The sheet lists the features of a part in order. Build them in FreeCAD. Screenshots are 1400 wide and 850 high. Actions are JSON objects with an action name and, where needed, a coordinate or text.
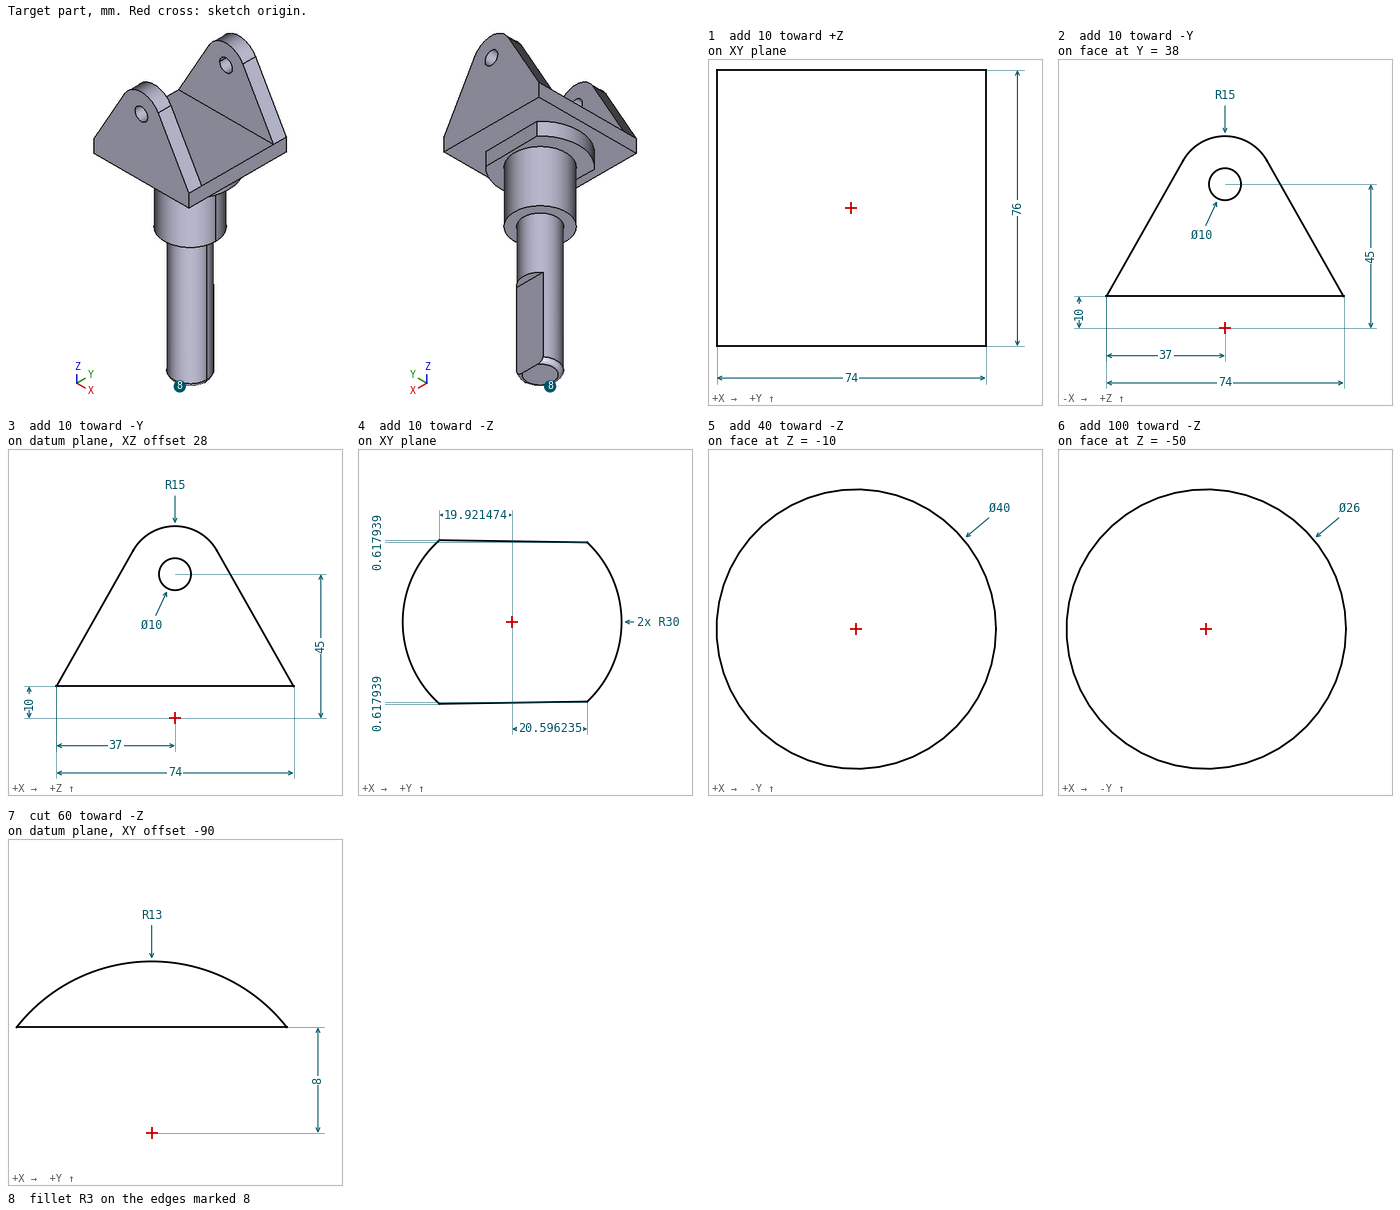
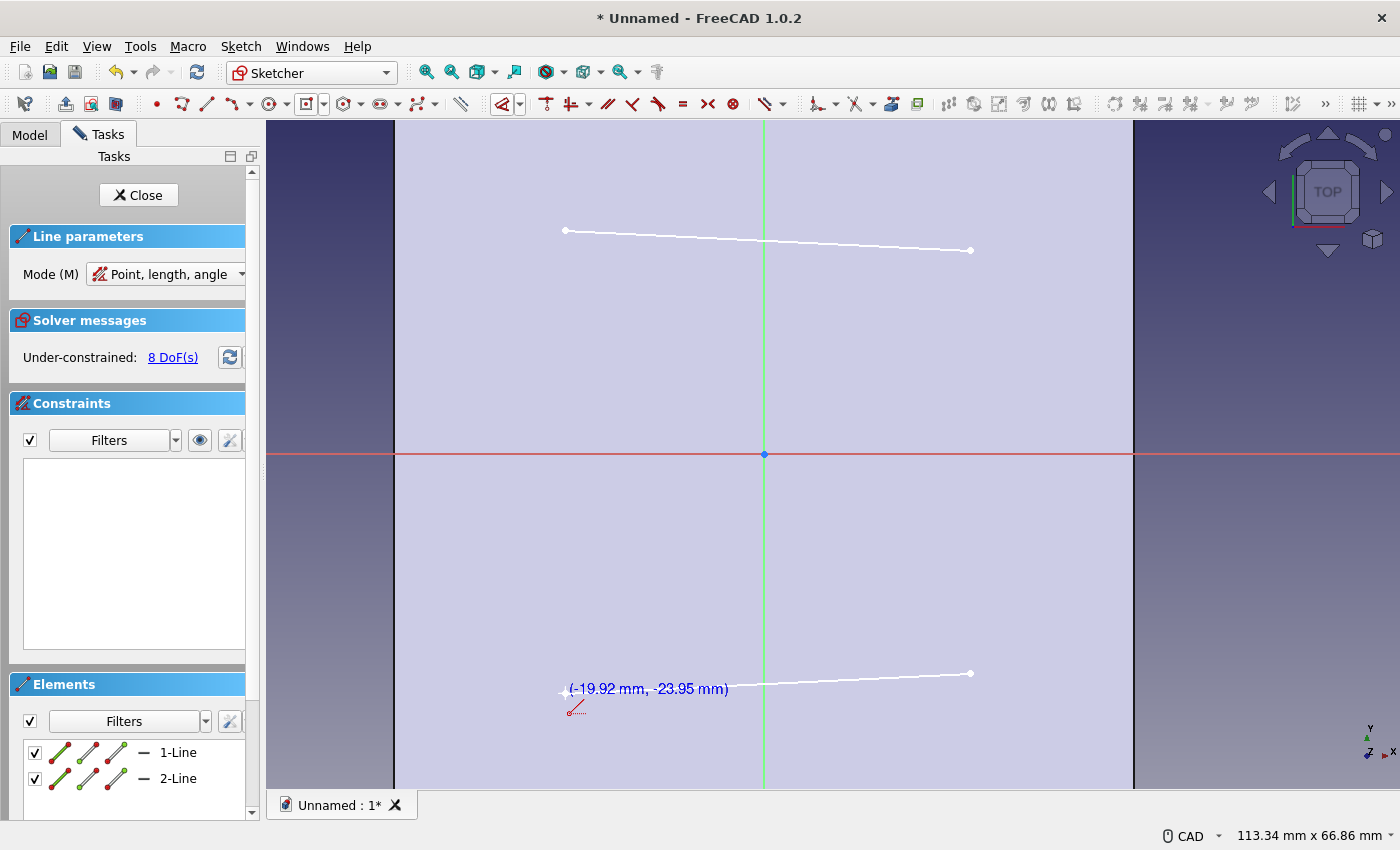
{"action": "left_click", "coordinate": [232, 104]}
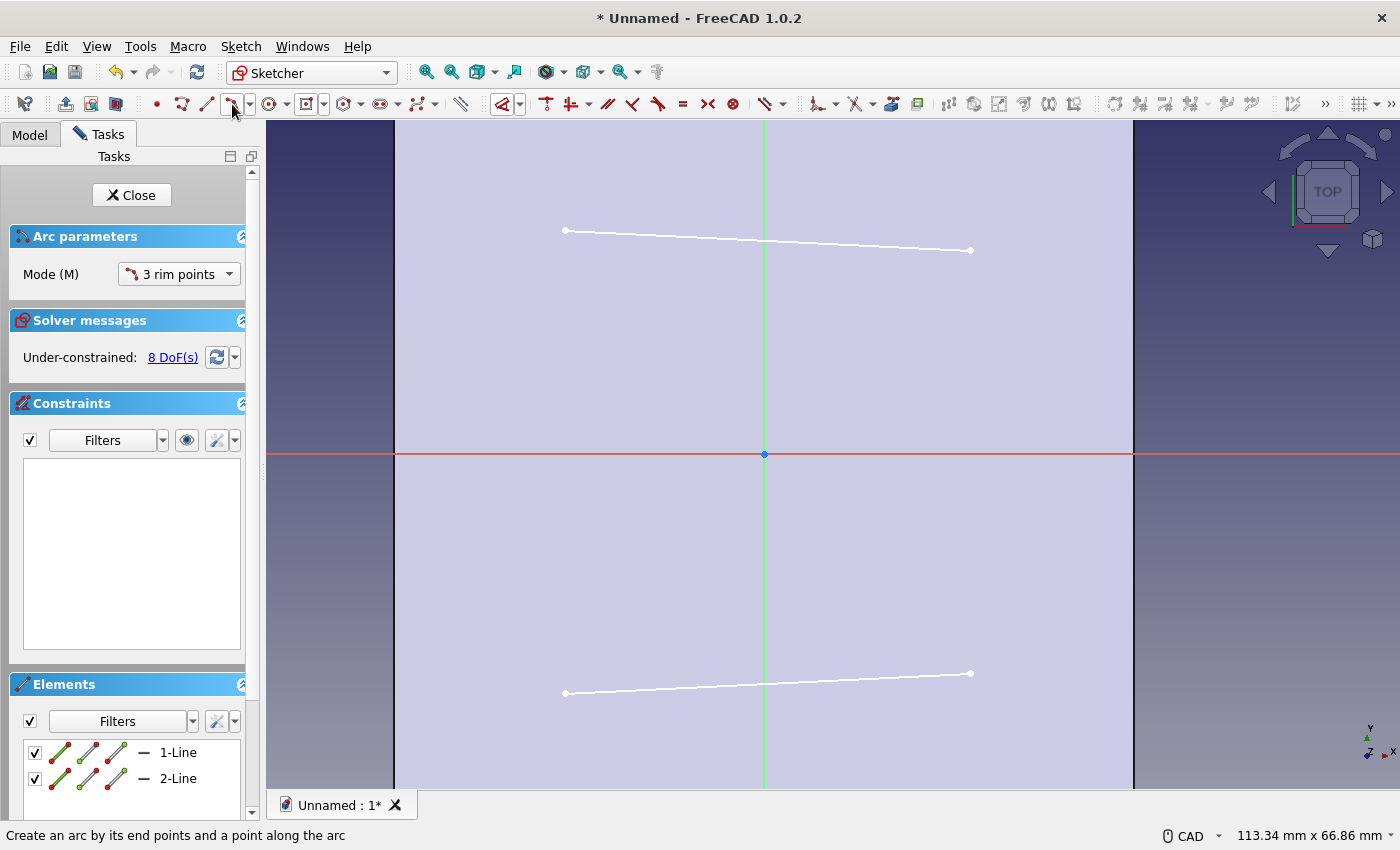
{"action": "left_click", "coordinate": [970, 251]}
{"action": "left_click", "coordinate": [970, 674]}
{"action": "left_click", "coordinate": [1060, 503]}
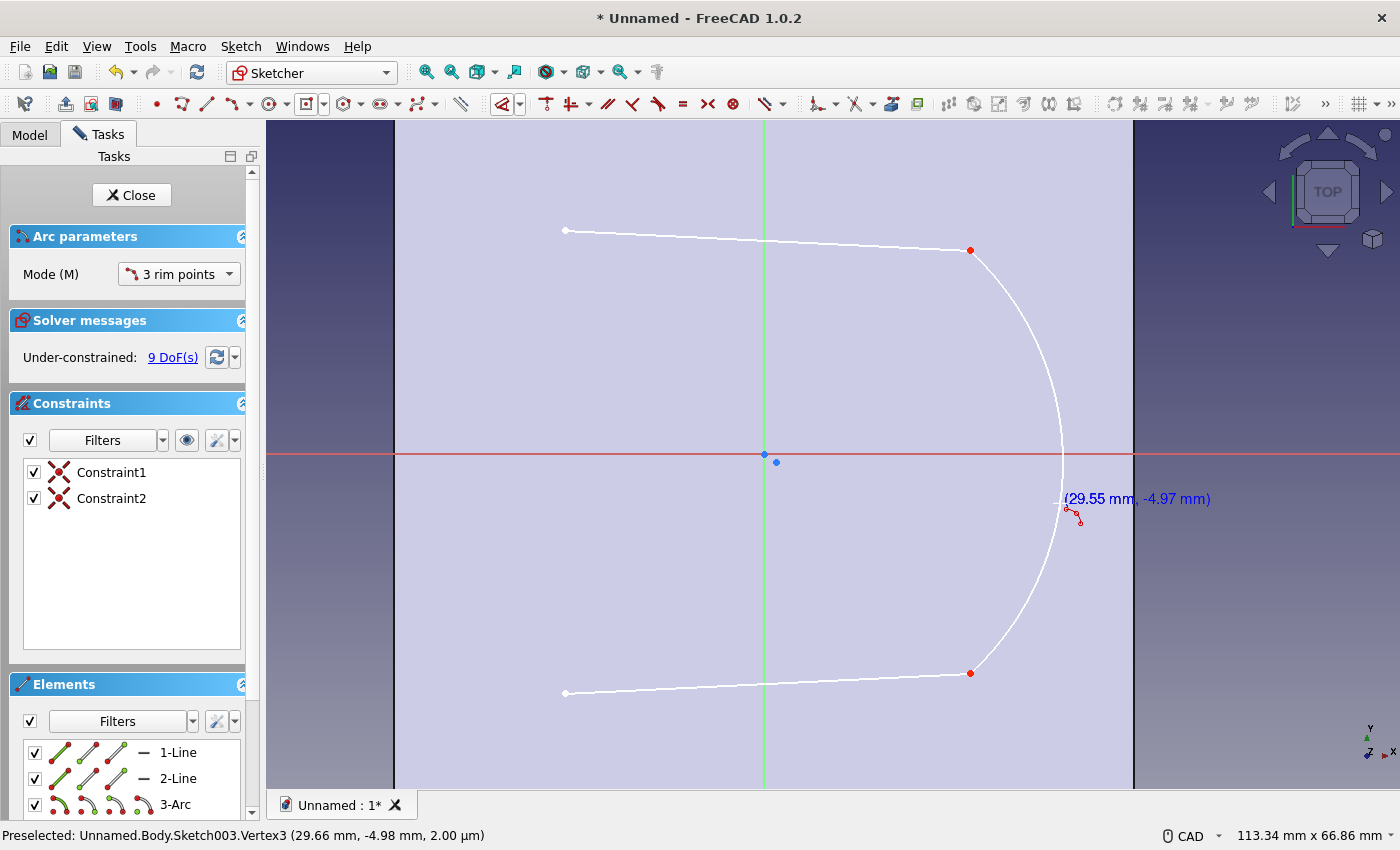
{"action": "left_click", "coordinate": [565, 694]}
{"action": "left_click", "coordinate": [565, 231]}
{"action": "left_click", "coordinate": [468, 404]}
{"action": "key", "text": "Escape"}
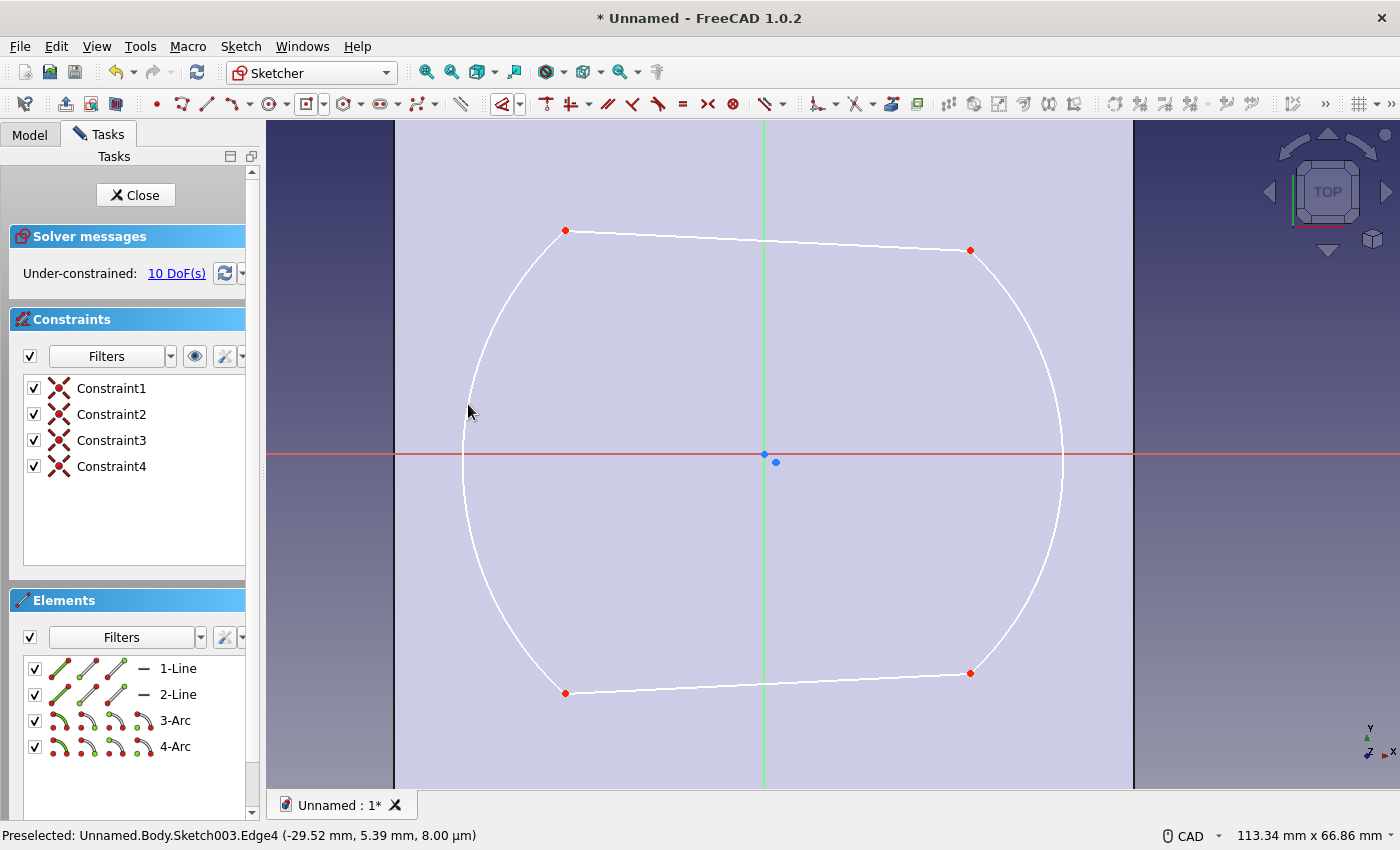
{"action": "left_click", "coordinate": [1047, 556]}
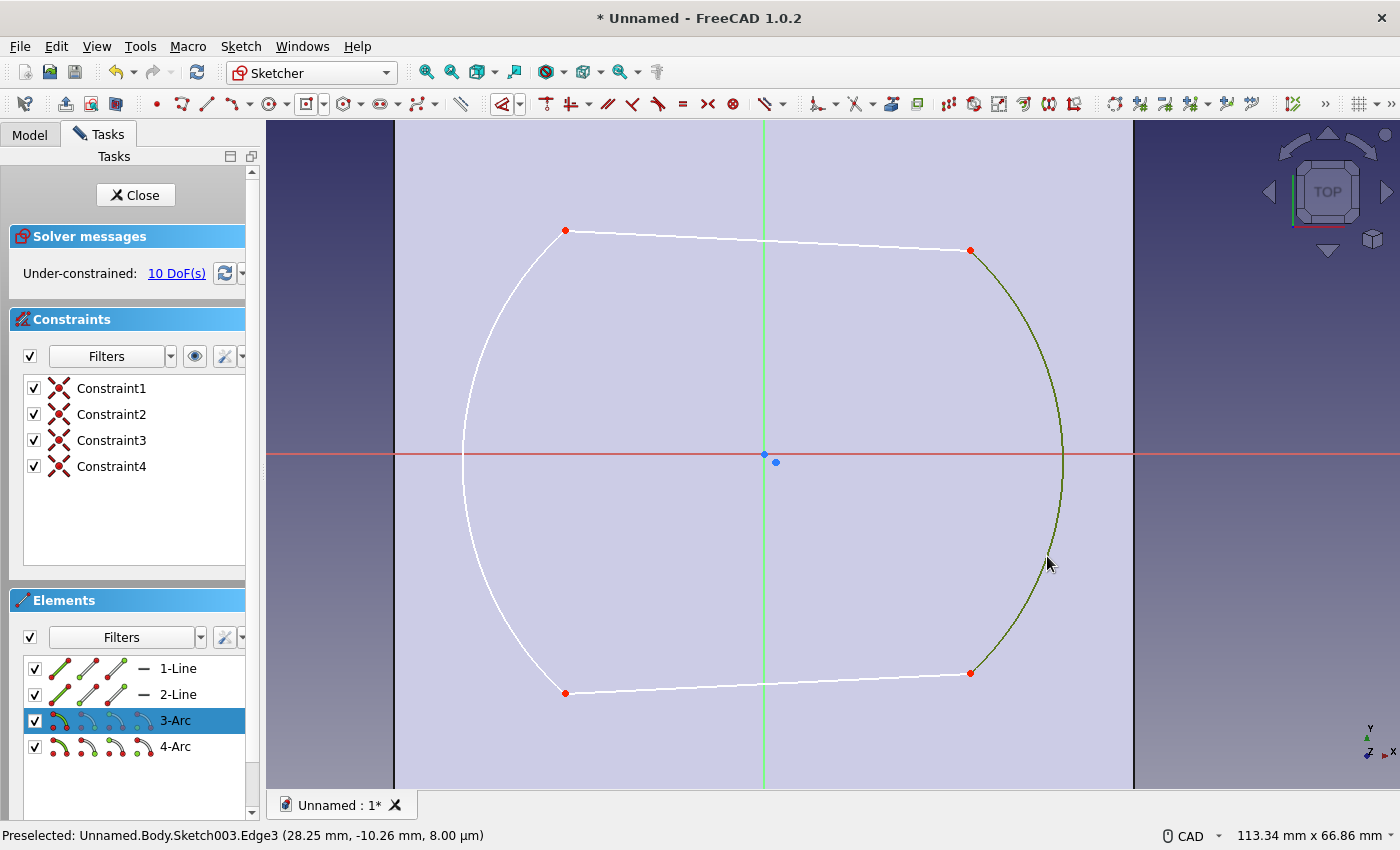
{"action": "left_click", "coordinate": [480, 360]}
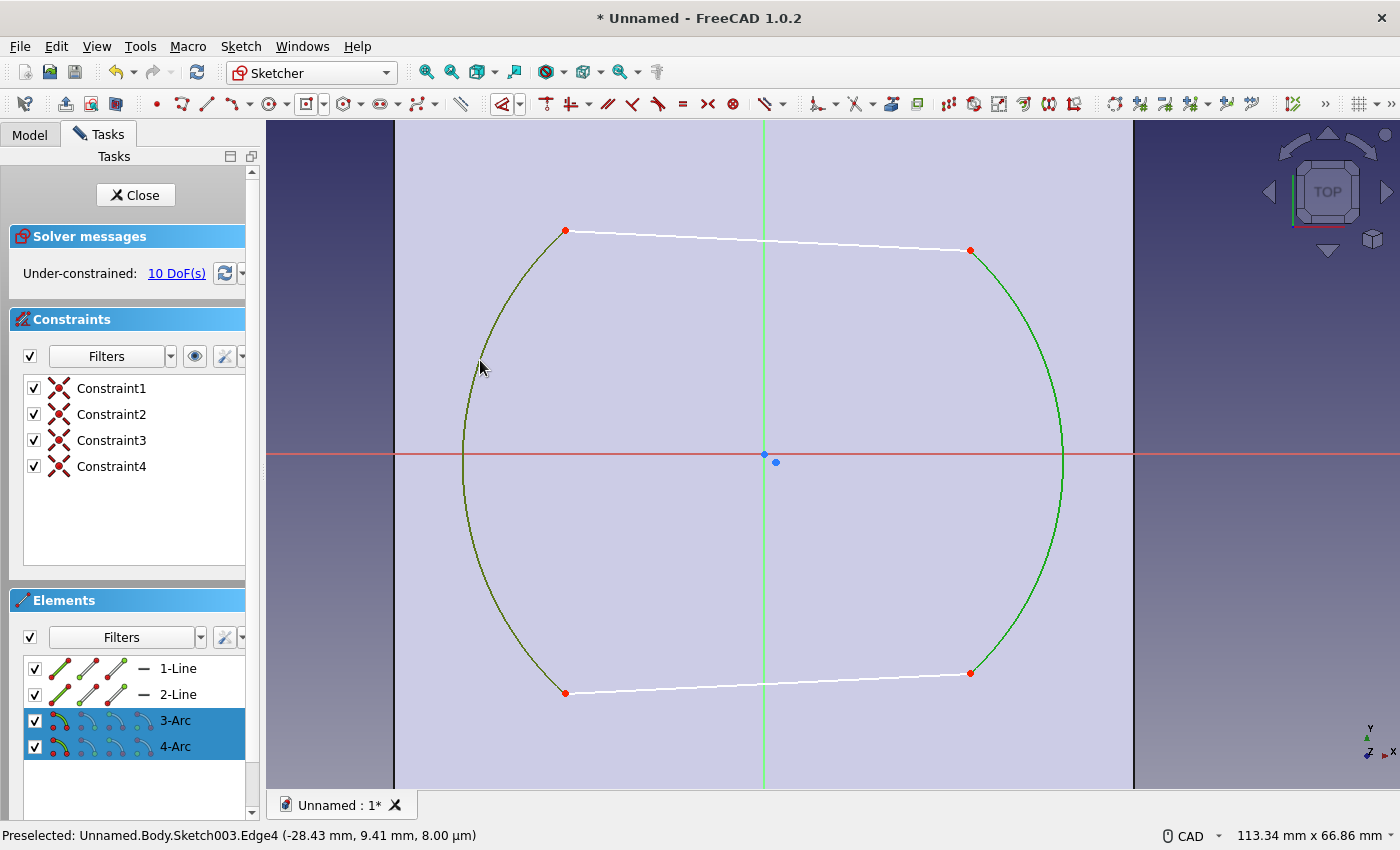
{"action": "left_click", "coordinate": [546, 104]}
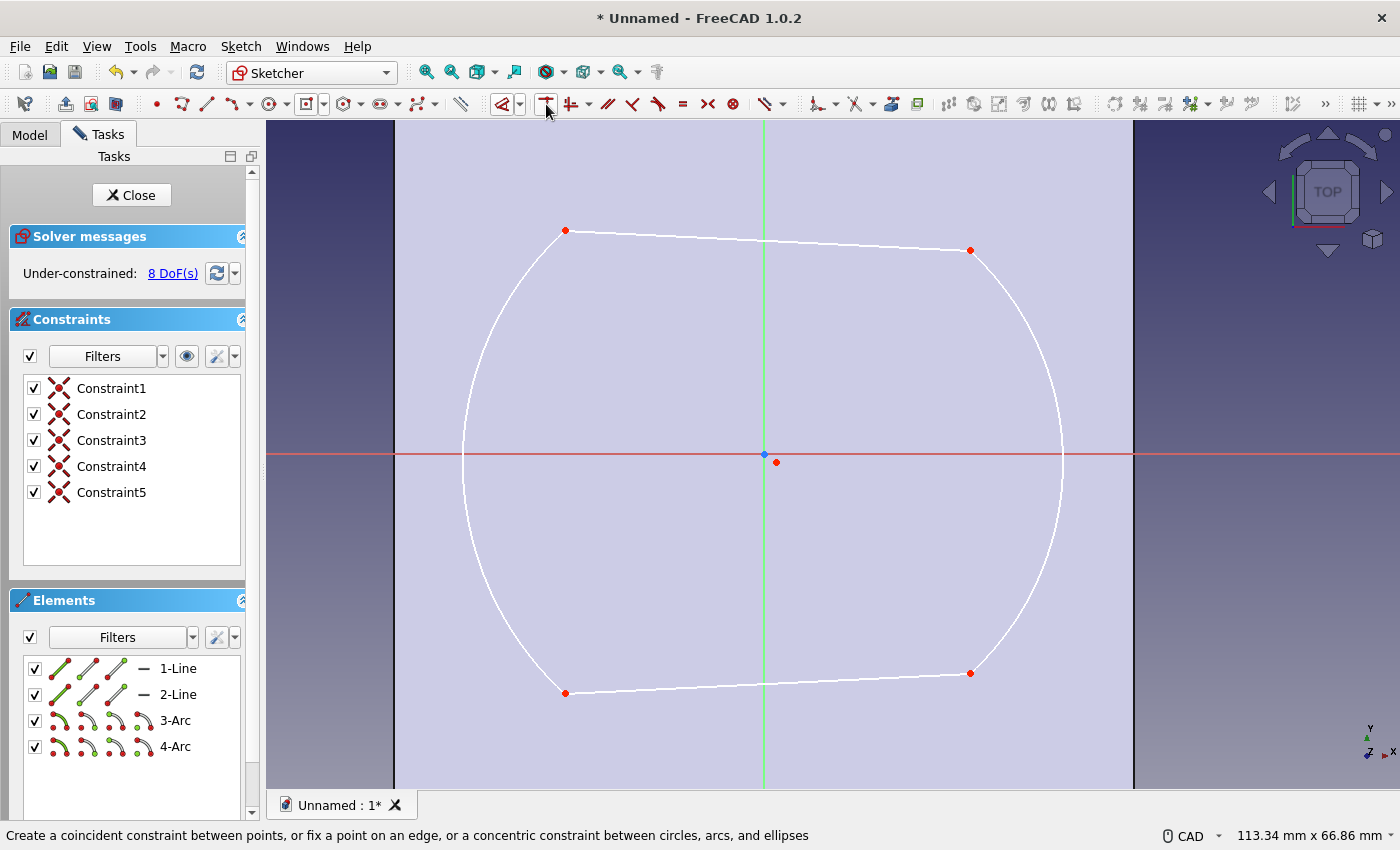
{"action": "left_click_drag", "start_coordinate": [754, 444], "coordinate": [786, 473]}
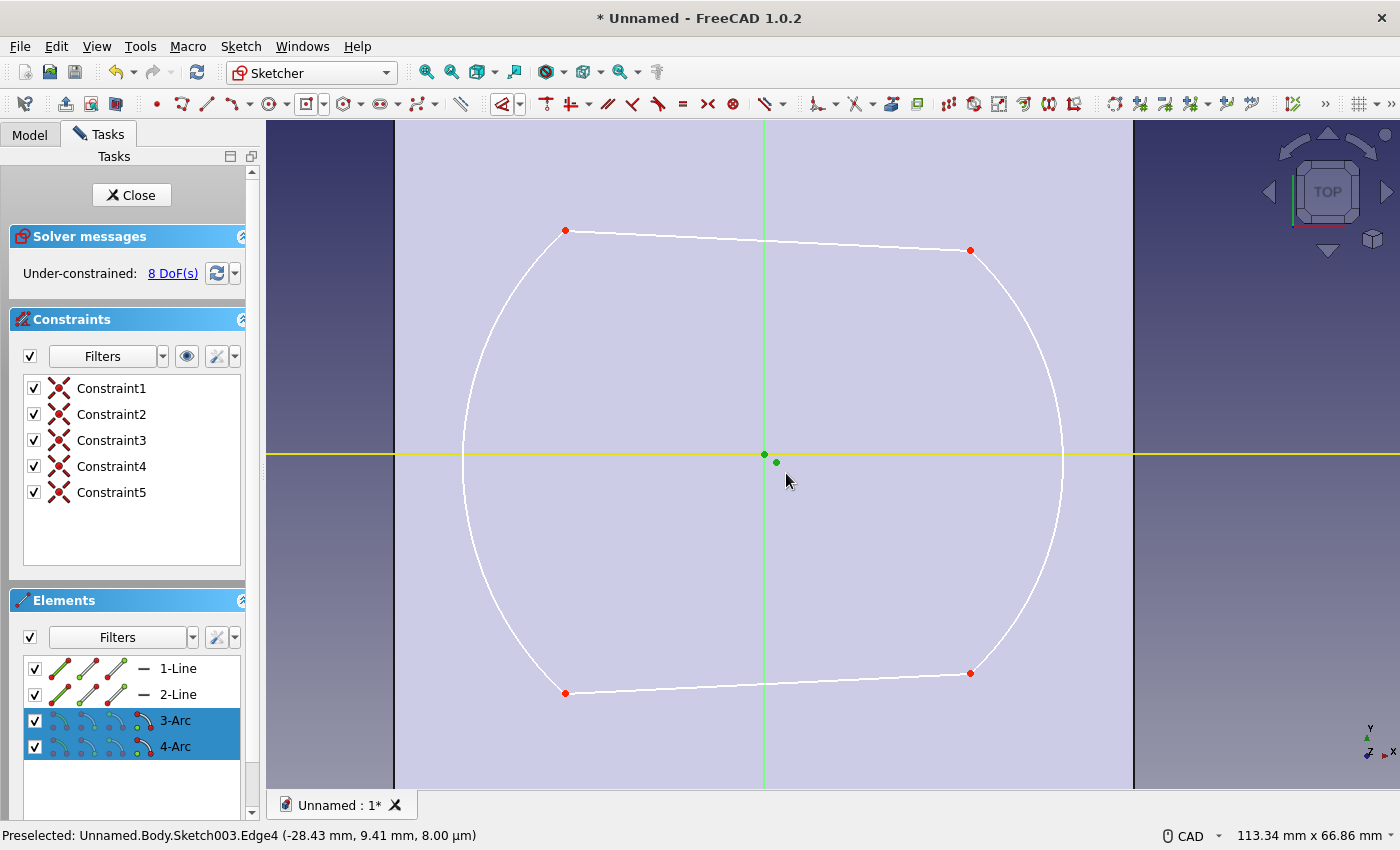
{"action": "left_click", "coordinate": [546, 104]}